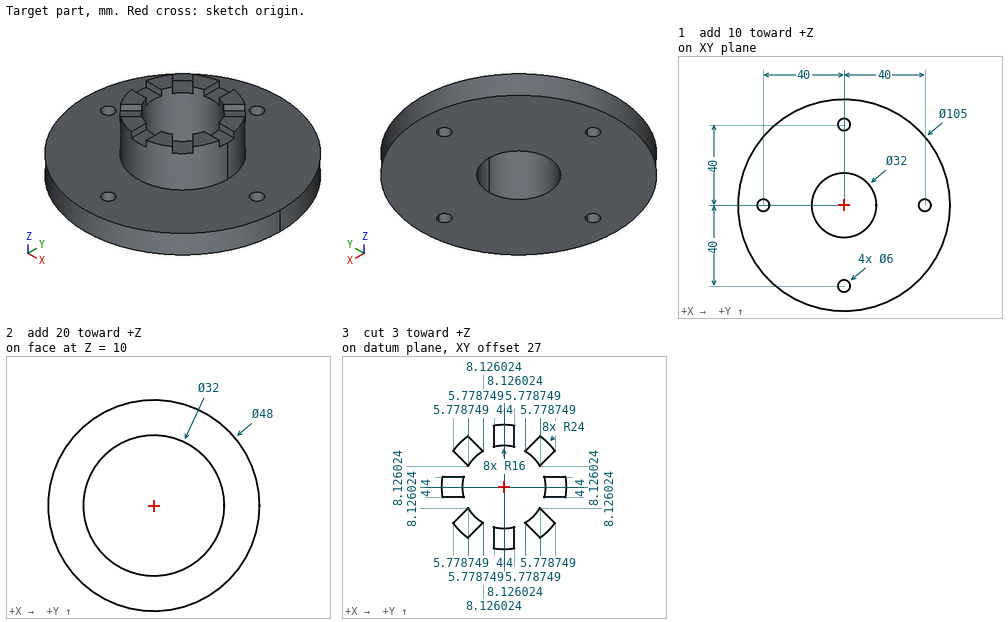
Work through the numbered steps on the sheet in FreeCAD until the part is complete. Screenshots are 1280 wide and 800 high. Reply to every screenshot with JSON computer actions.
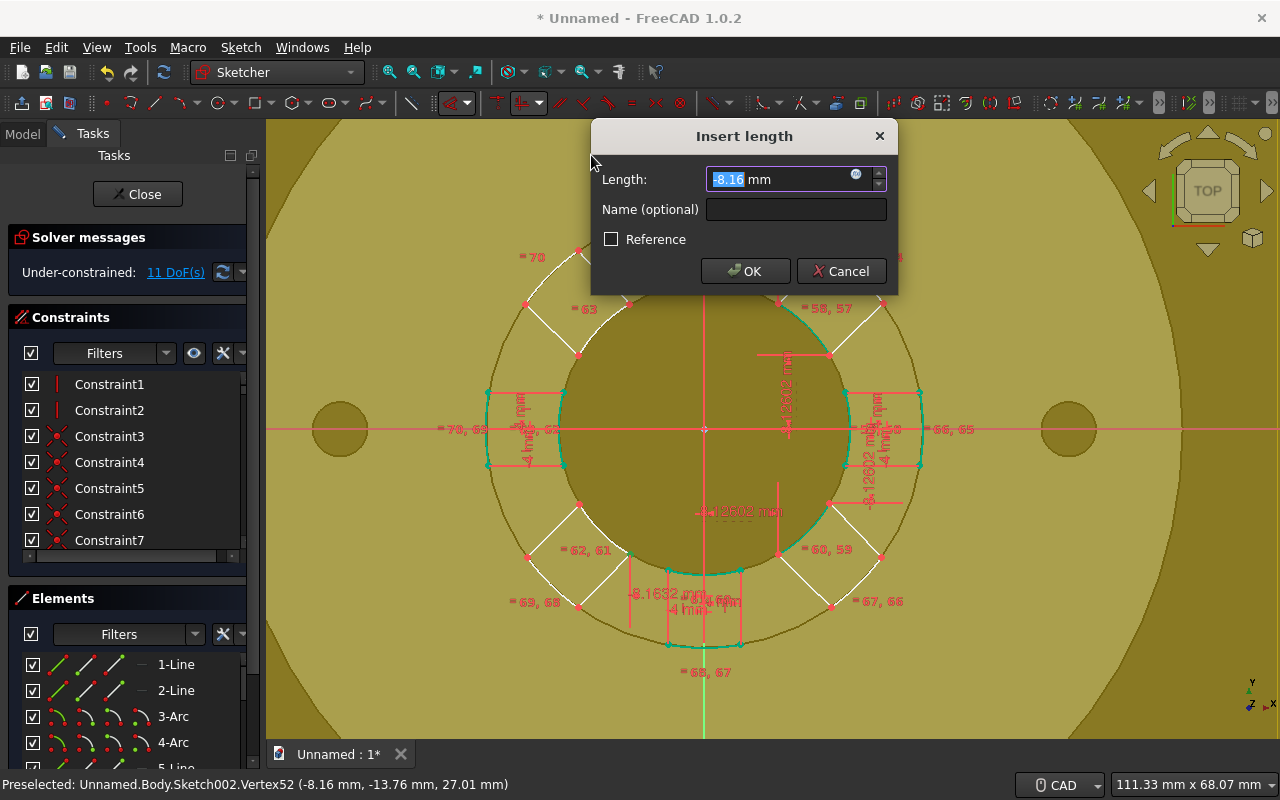
{"action": "type", "text": "-8.126024"}
{"action": "key", "text": "Return"}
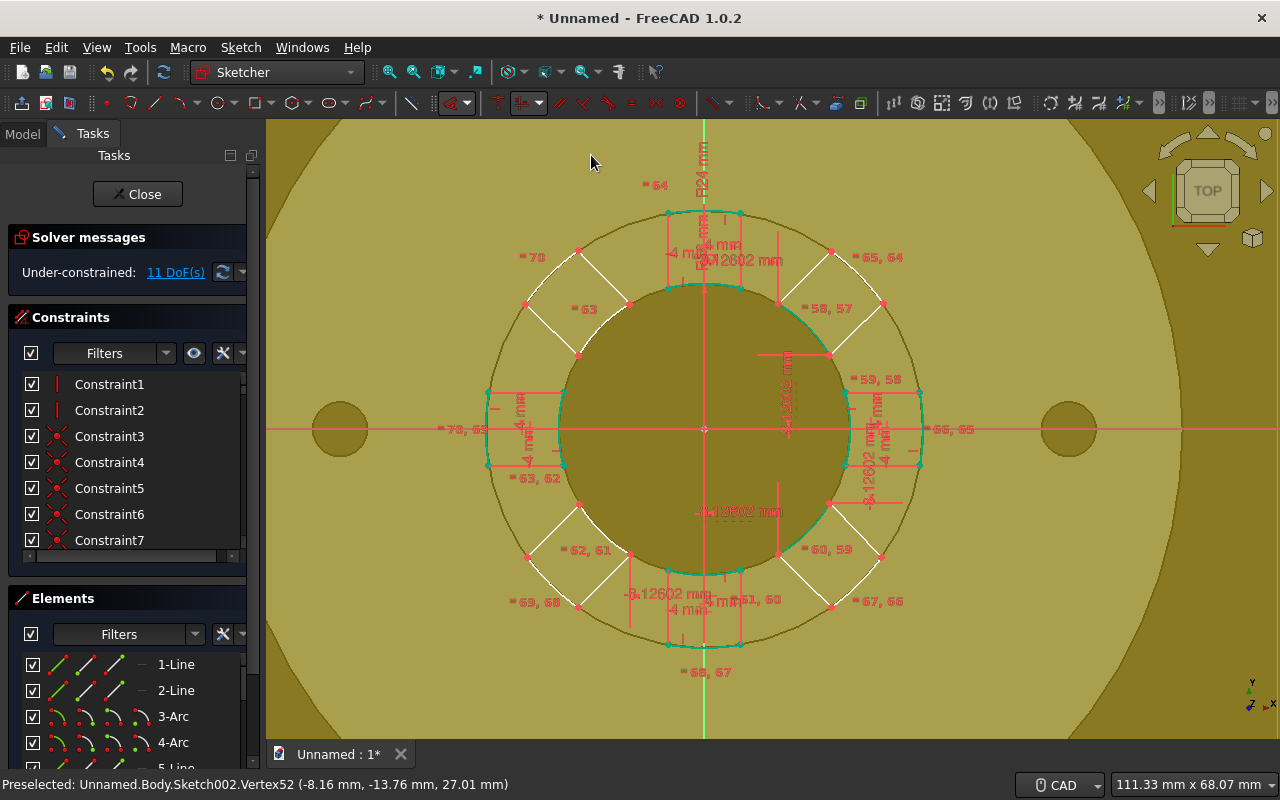
{"action": "left_click", "coordinate": [580, 504]}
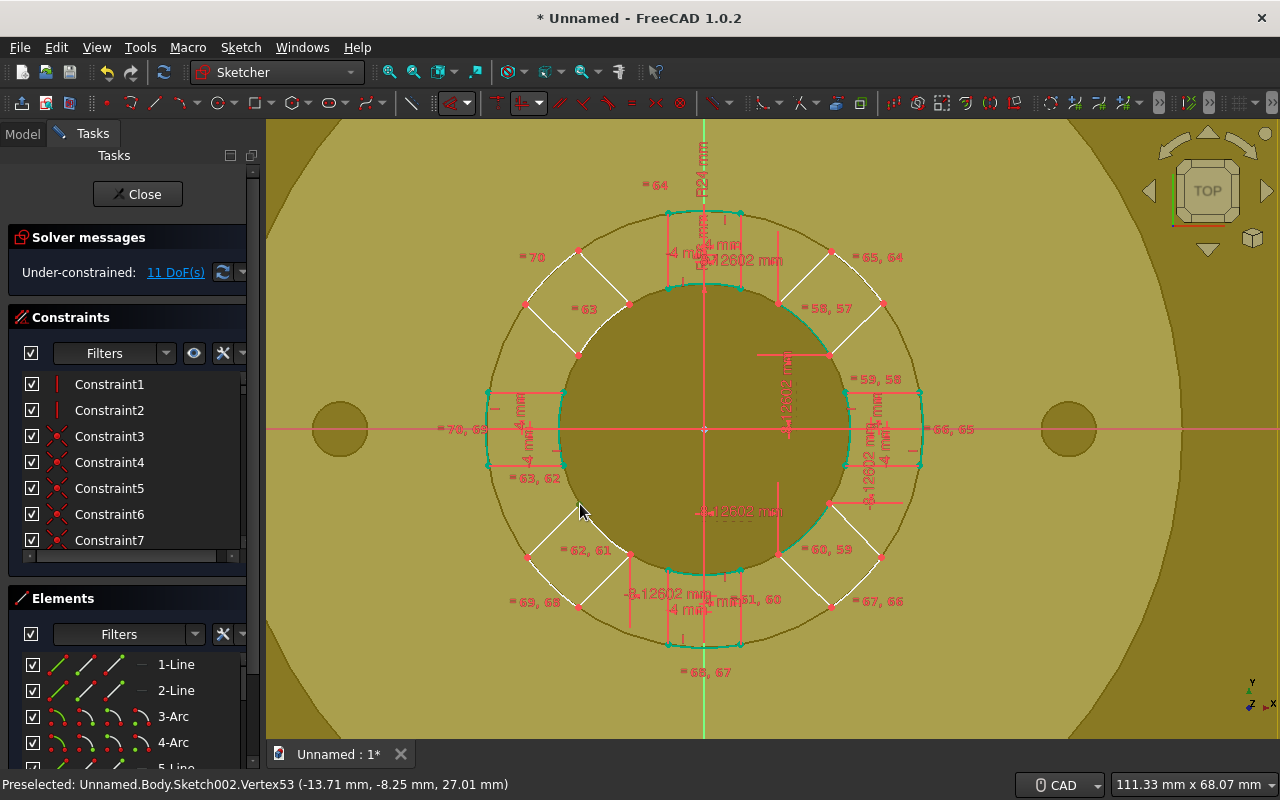
{"action": "left_click", "coordinate": [470, 104]}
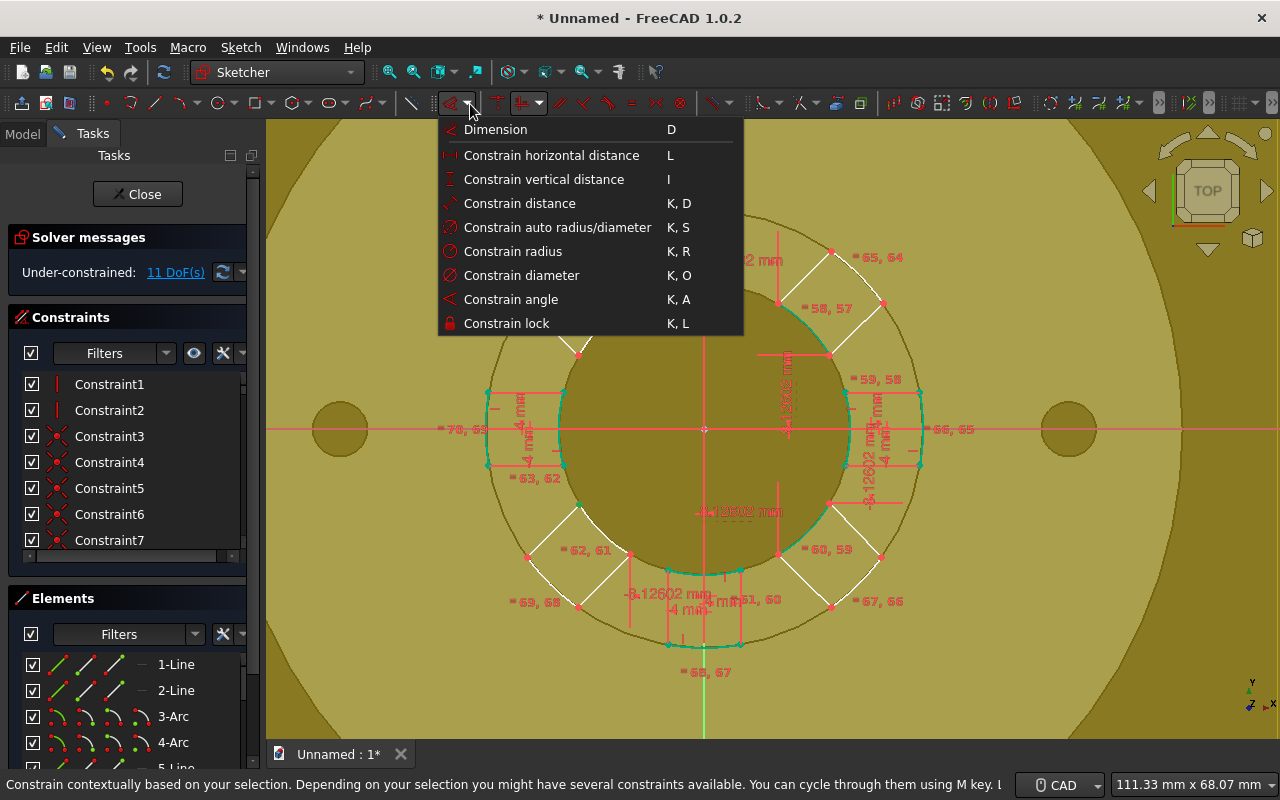
{"action": "left_click", "coordinate": [591, 179]}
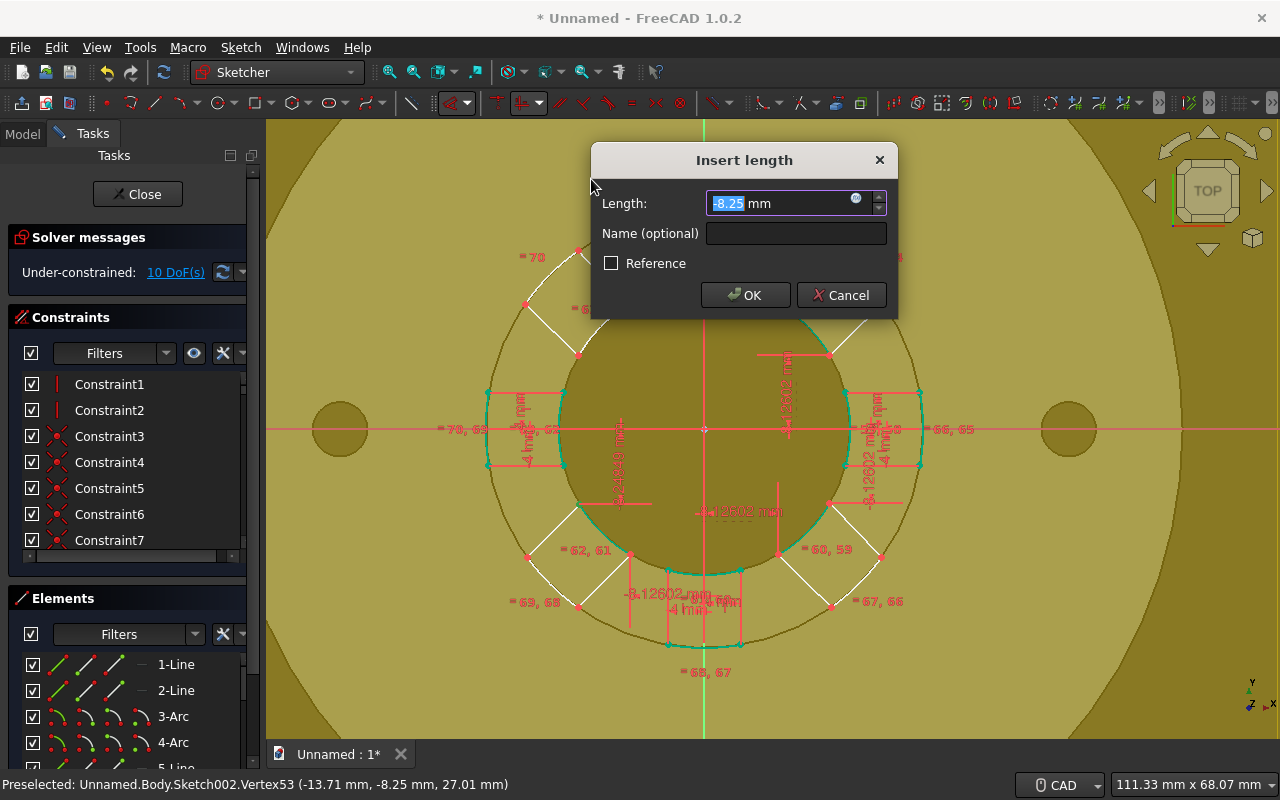
{"action": "type", "text": "-8.126024"}
{"action": "key", "text": "Return"}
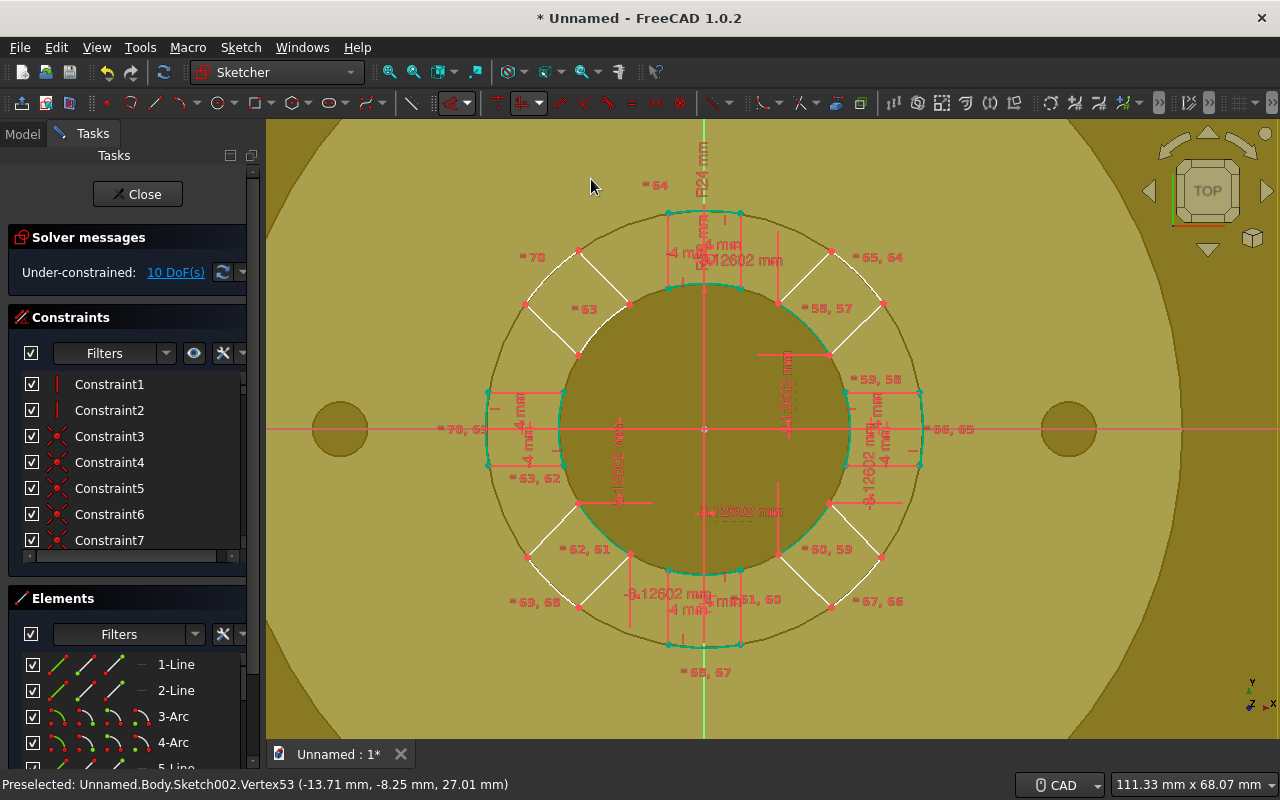
{"action": "left_click", "coordinate": [579, 356]}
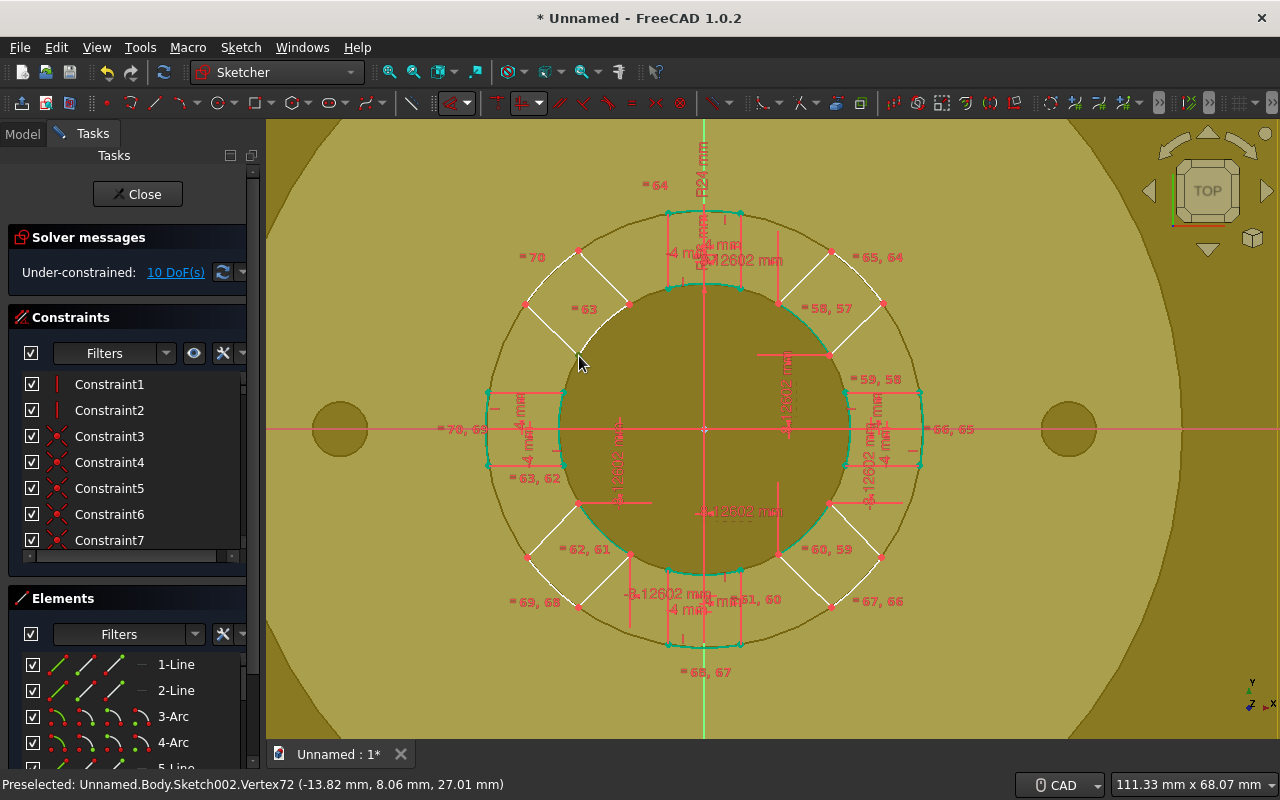
{"action": "left_click", "coordinate": [470, 104]}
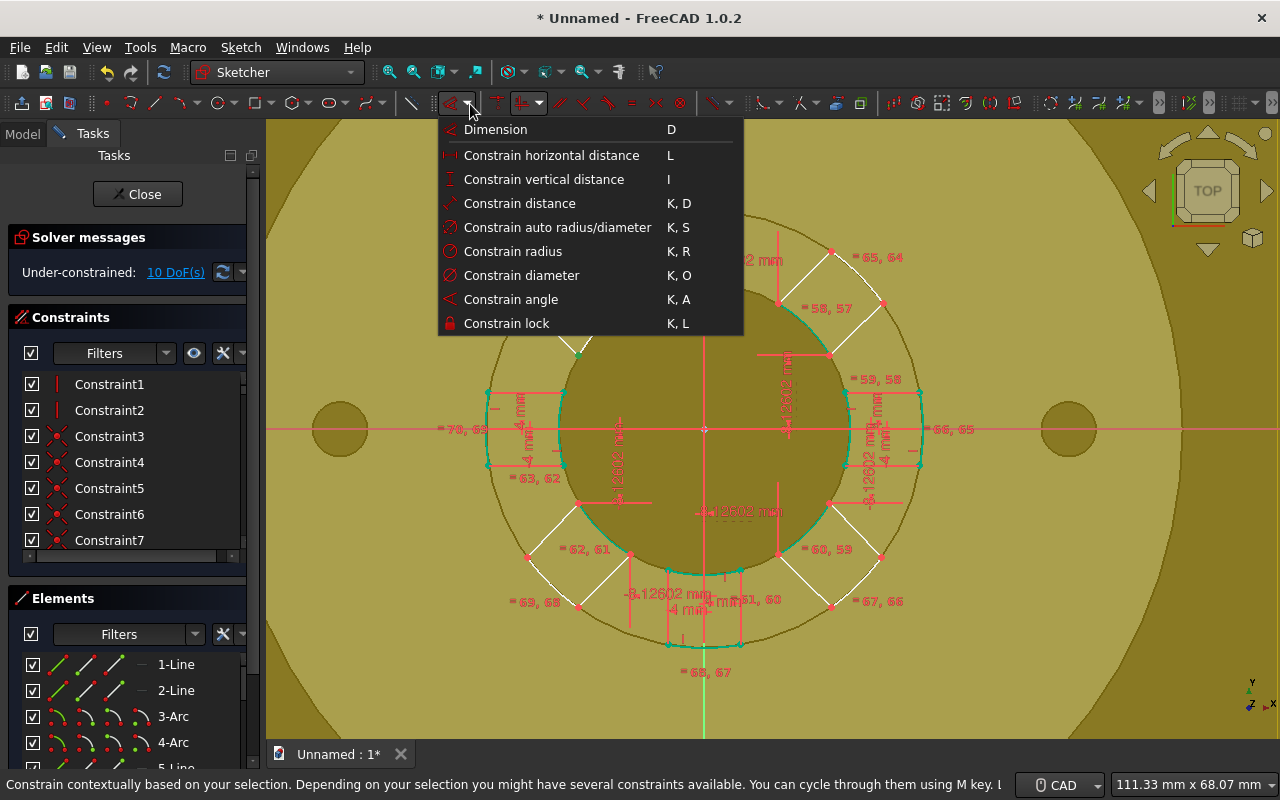
{"action": "left_click", "coordinate": [591, 179]}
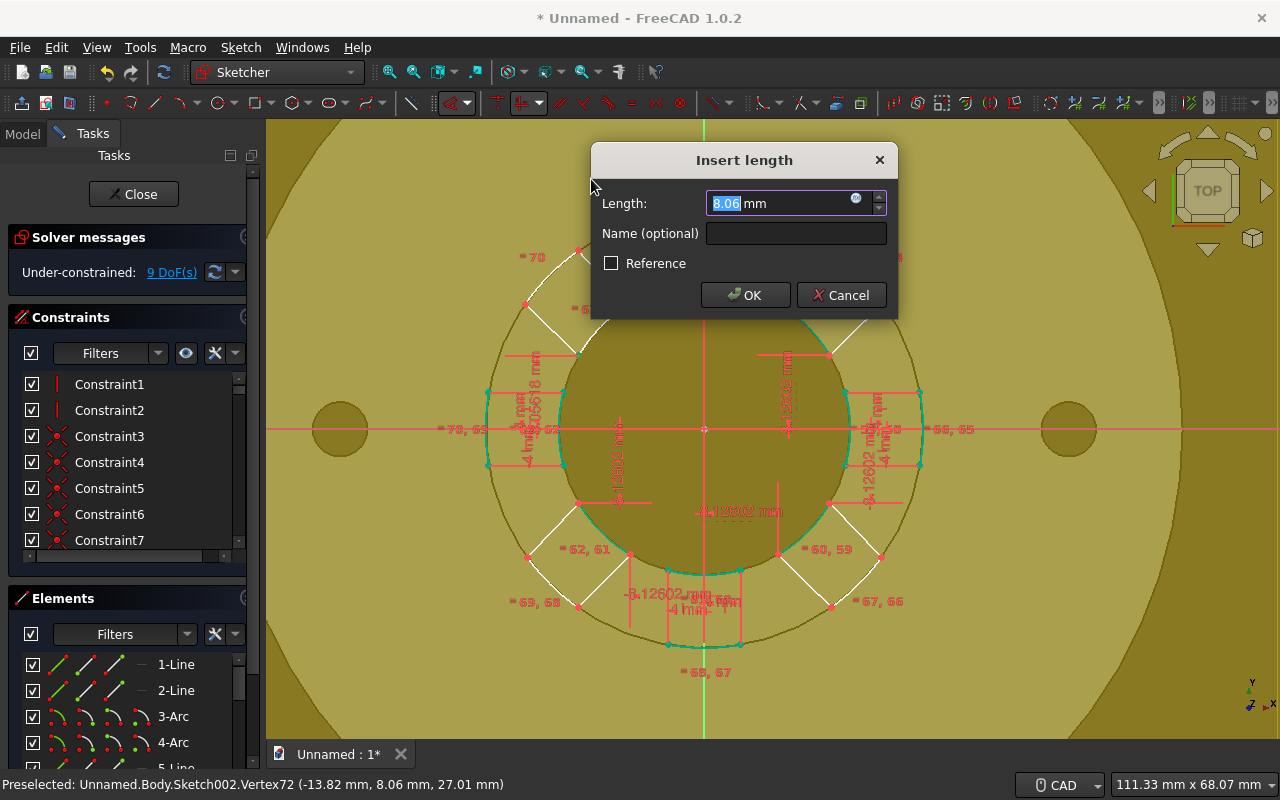
{"action": "type", "text": "8.126024"}
{"action": "key", "text": "Return"}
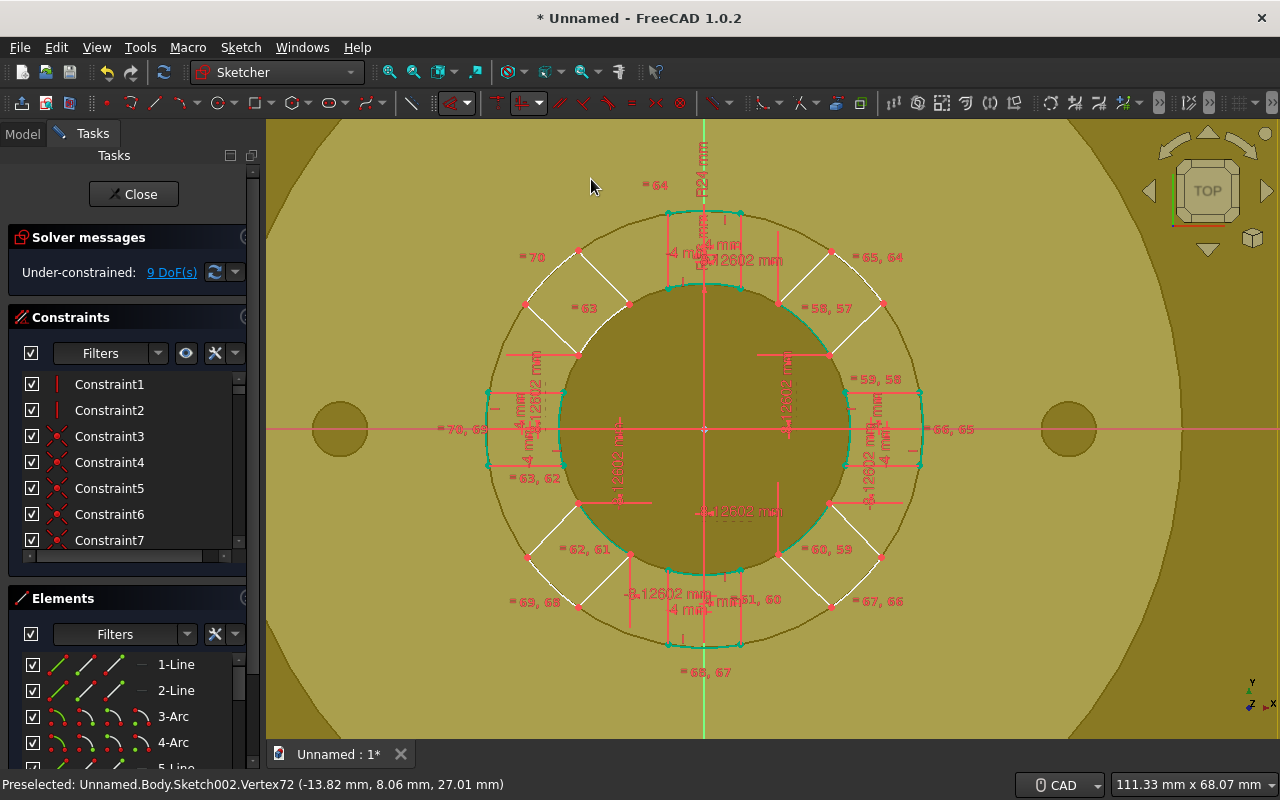
{"action": "left_click", "coordinate": [630, 304]}